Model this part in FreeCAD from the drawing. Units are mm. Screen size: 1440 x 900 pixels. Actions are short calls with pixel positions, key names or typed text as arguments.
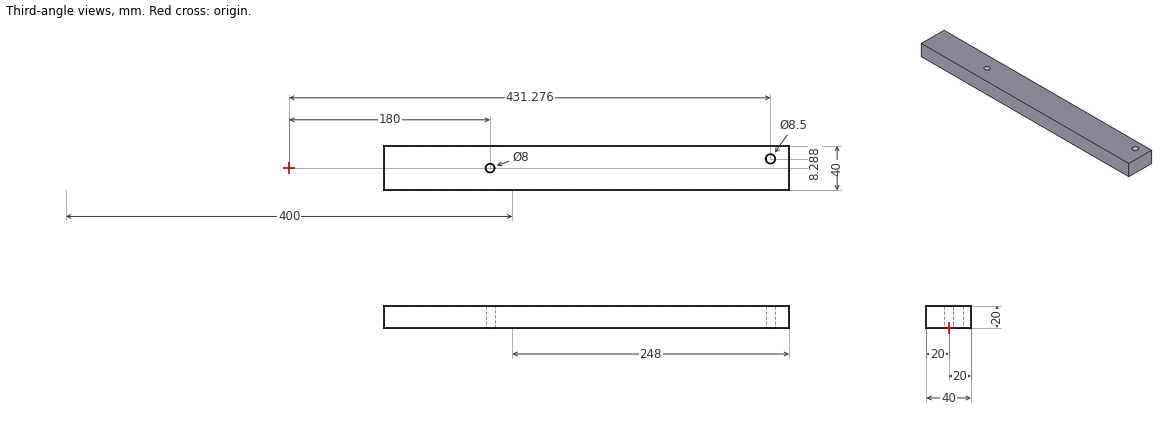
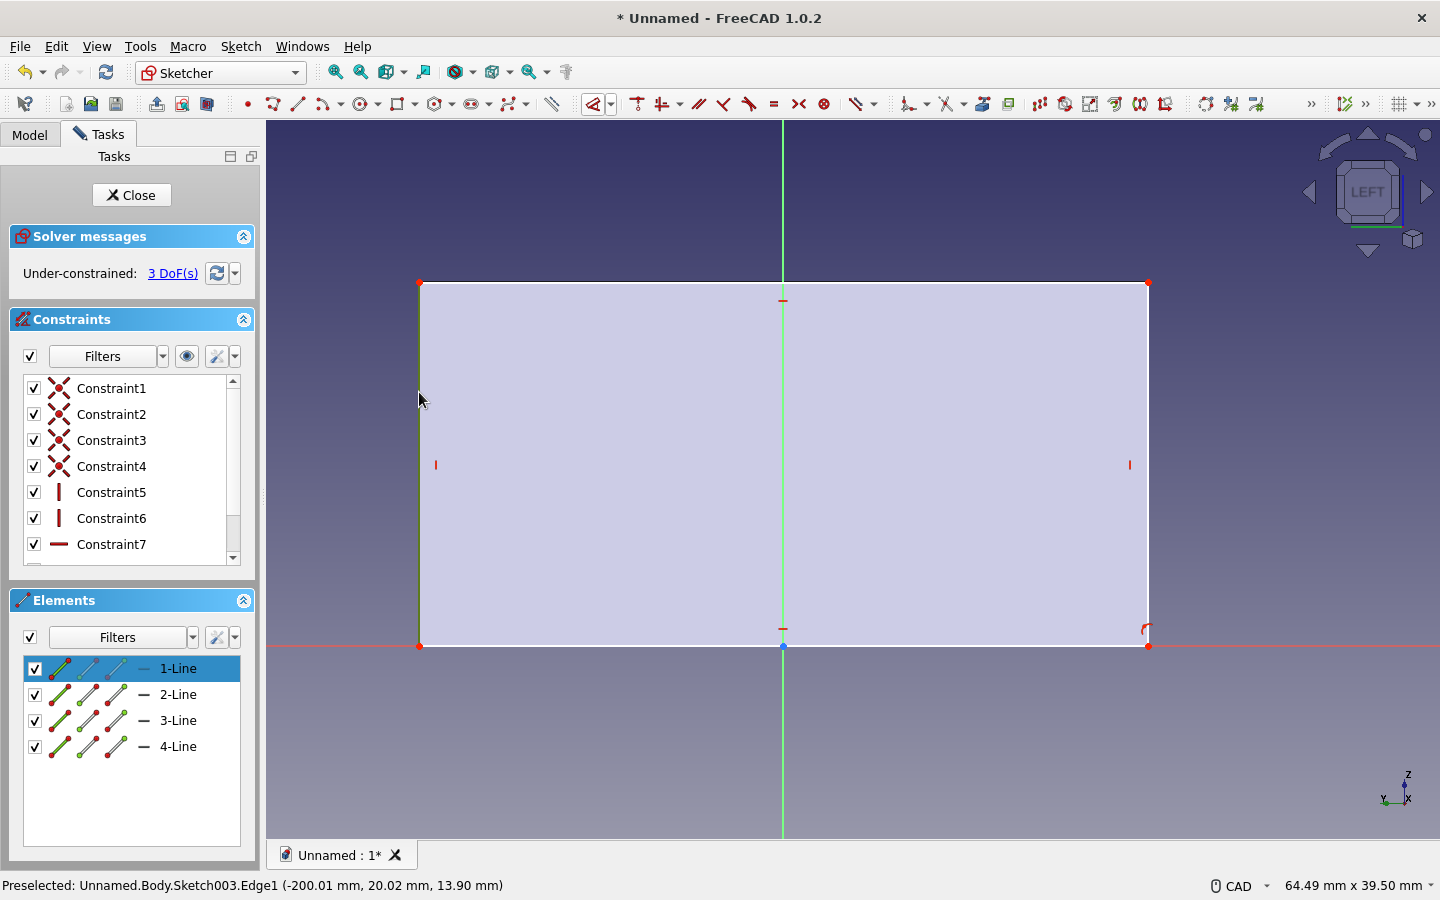
click(610, 104)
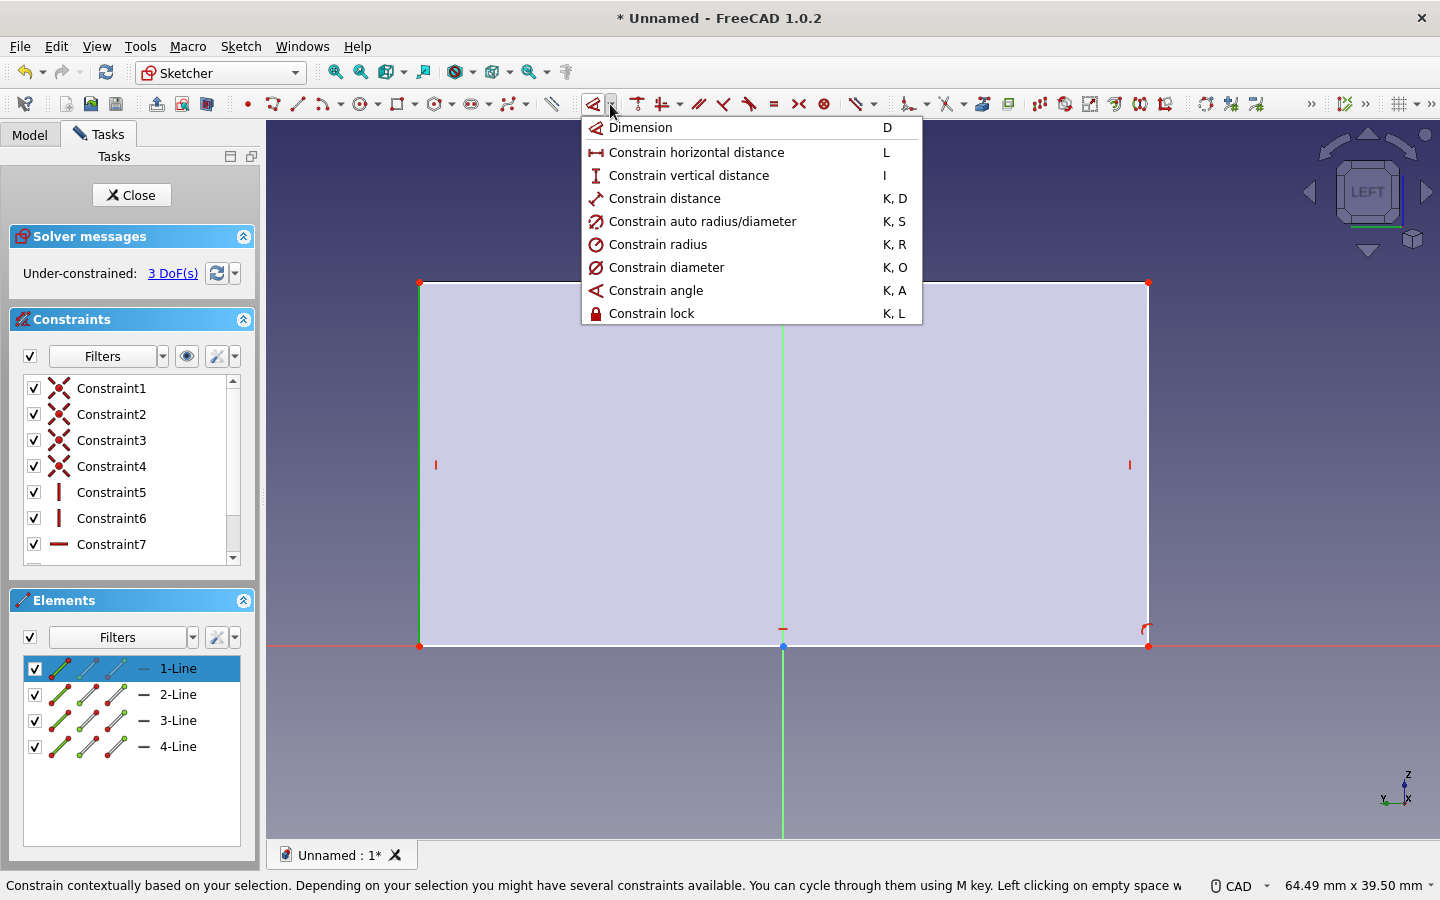
click(752, 176)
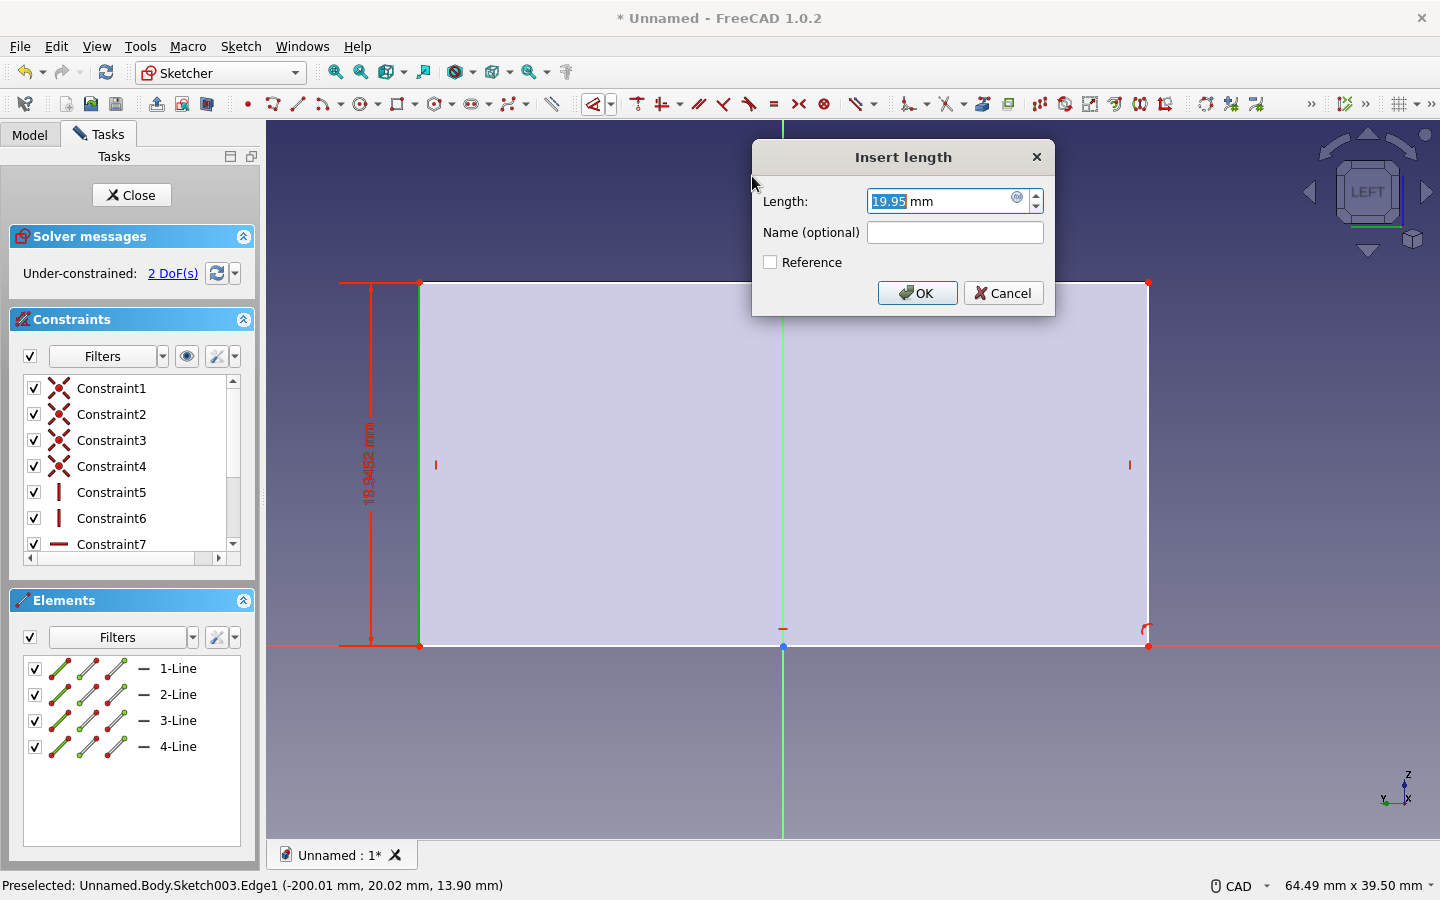
text(20)
key(Return)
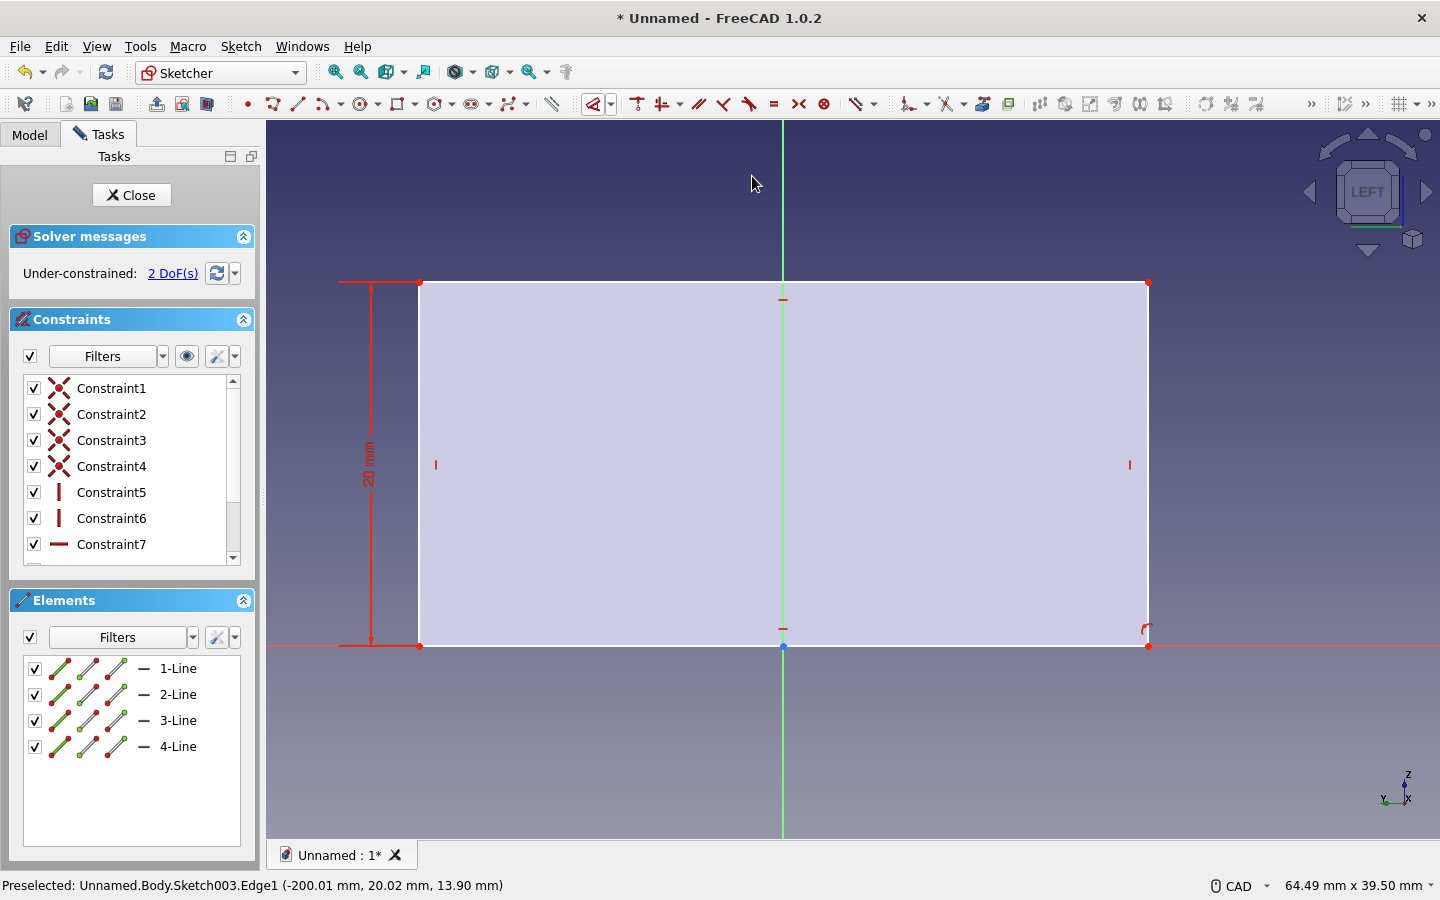
click(638, 646)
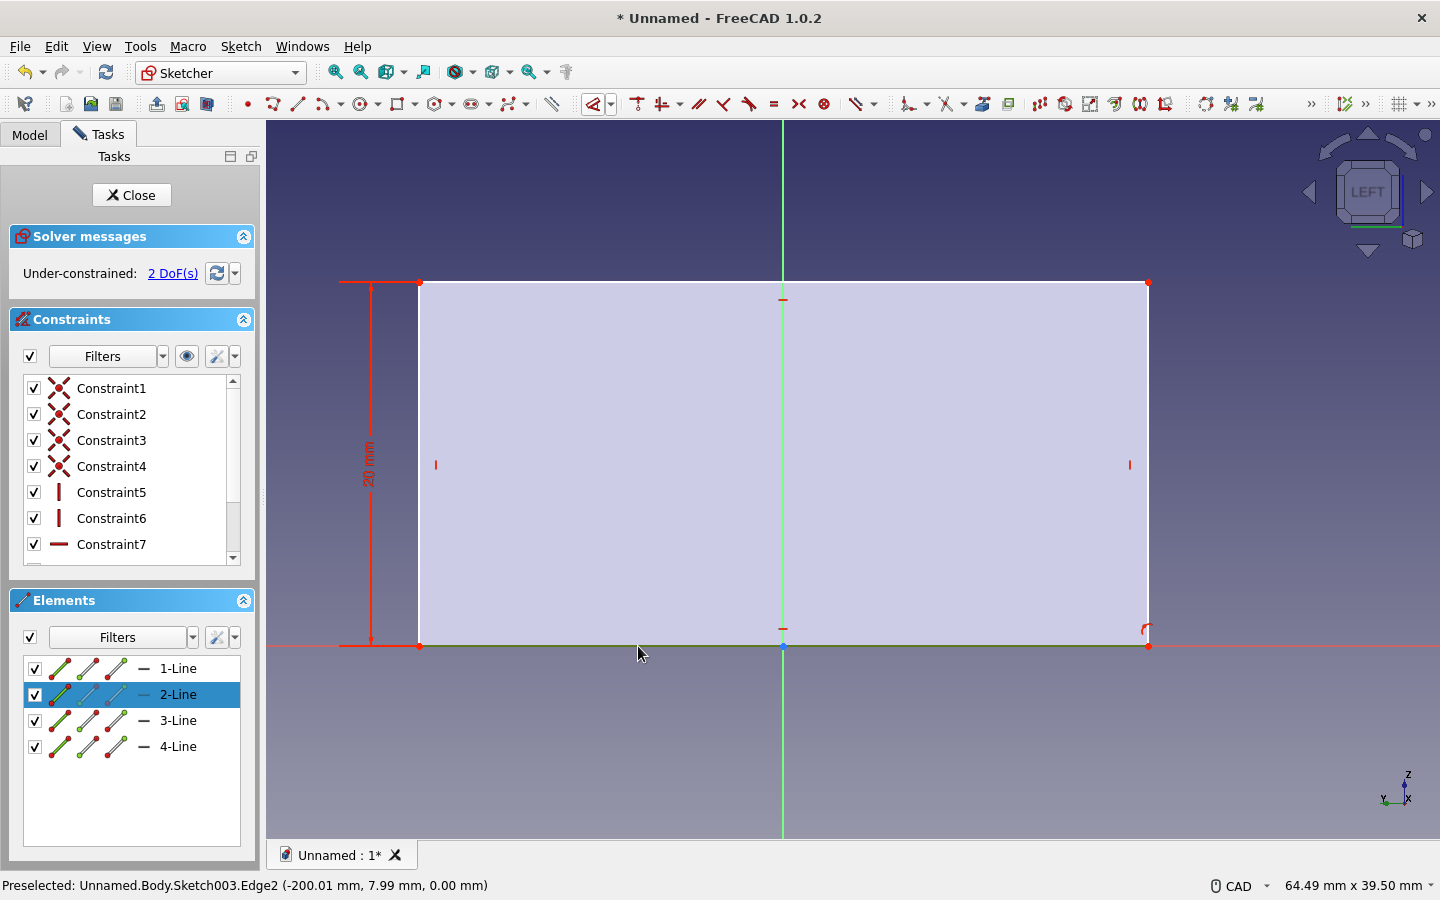
click(610, 104)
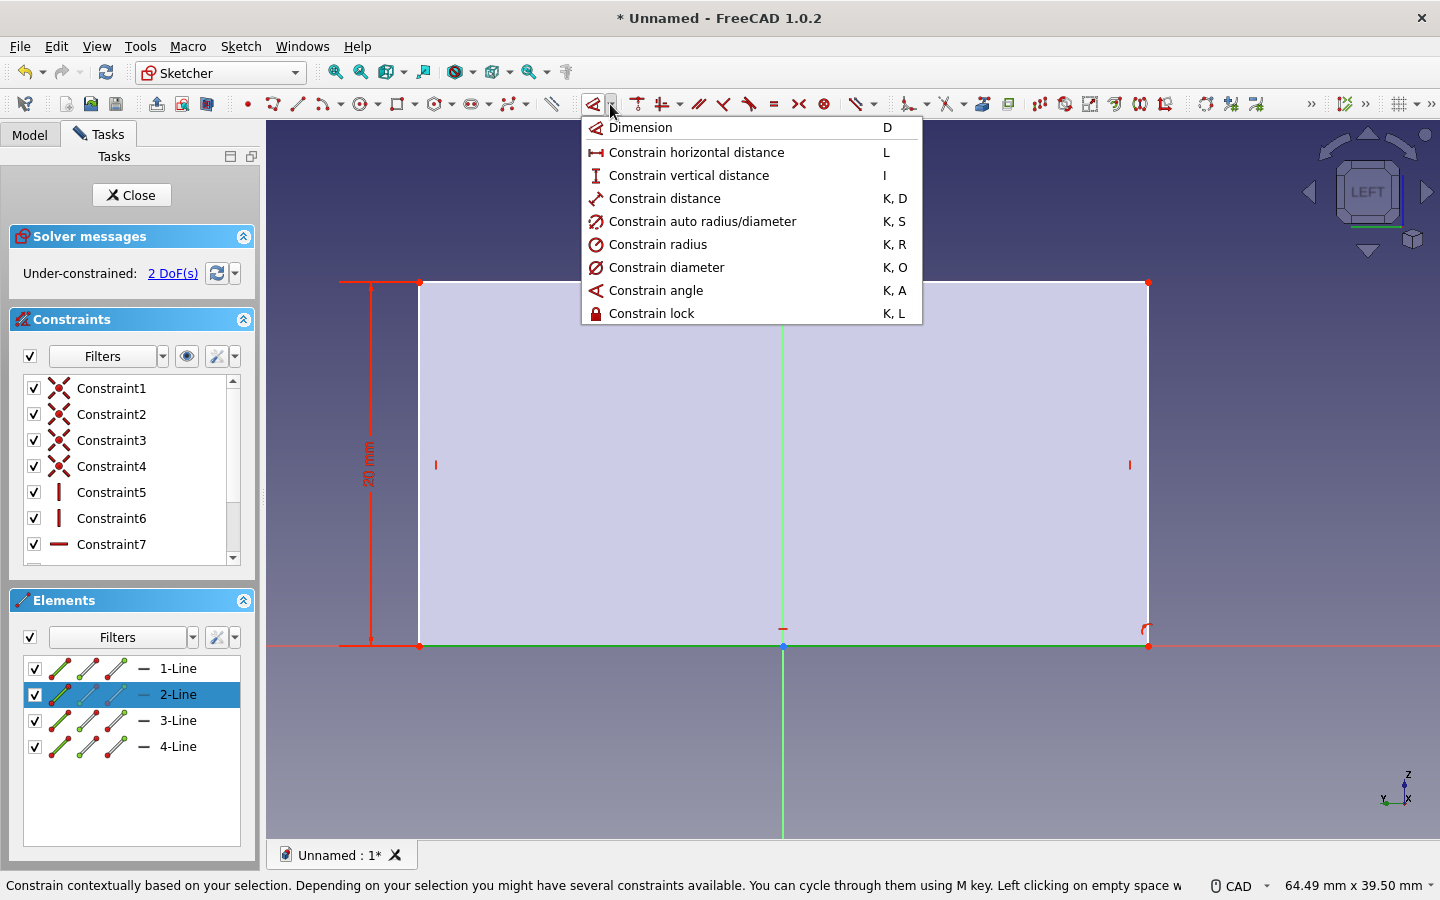
click(752, 152)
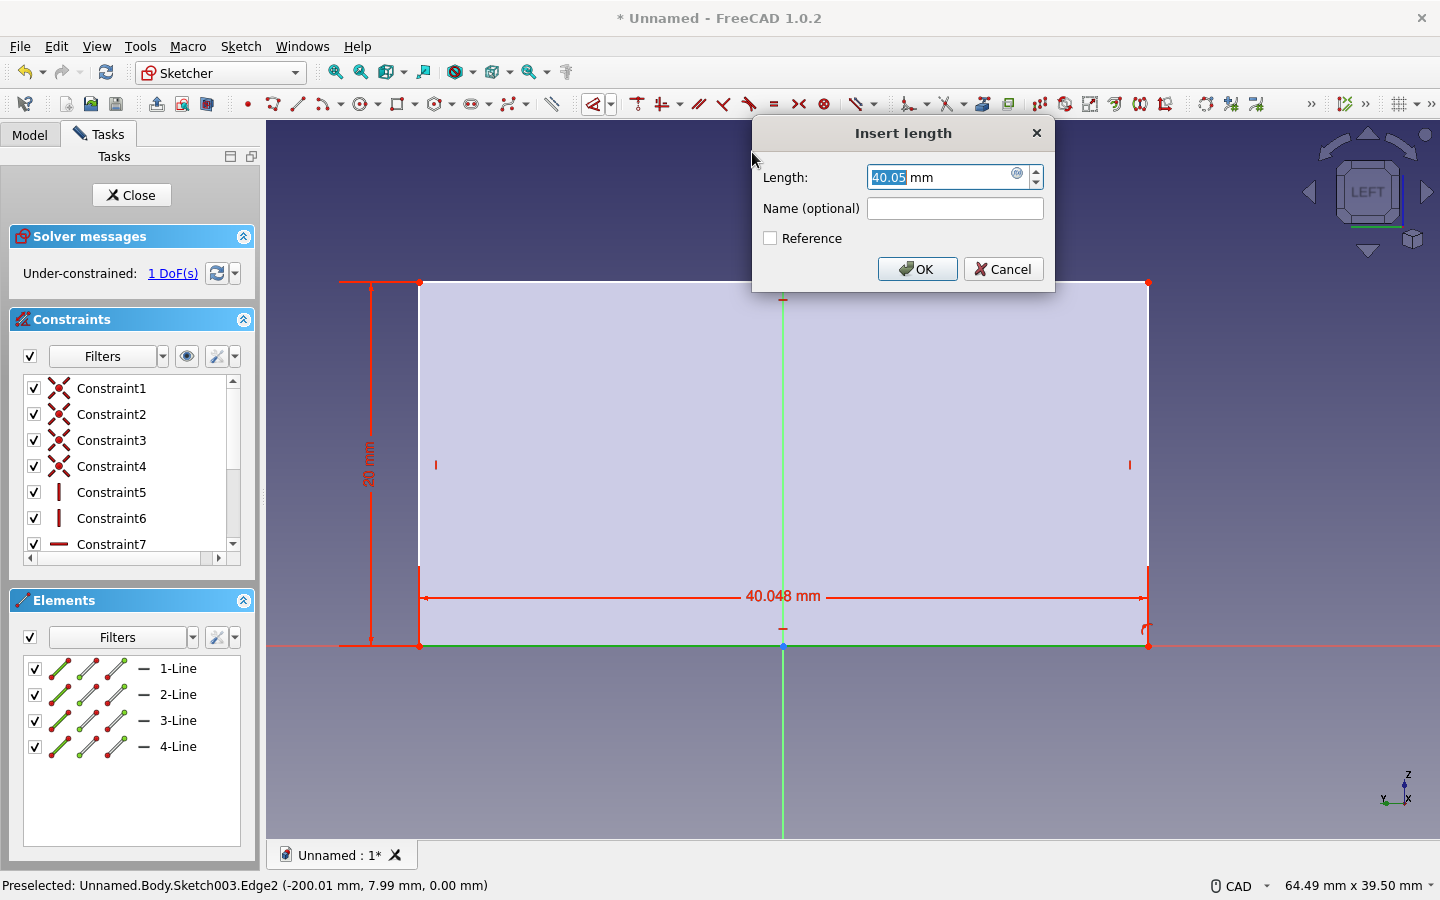
text(40)
key(Return)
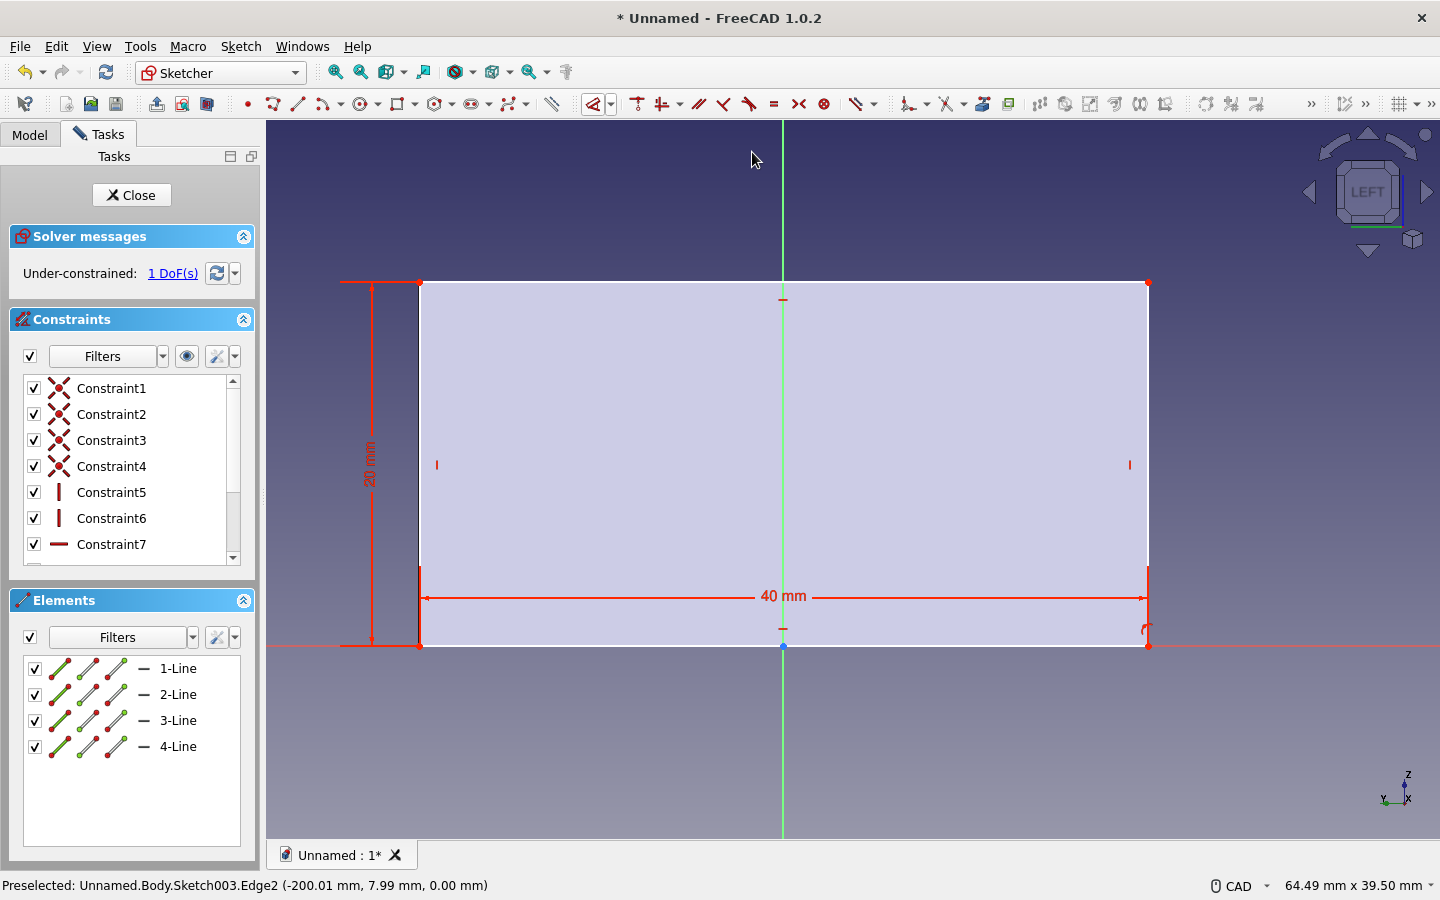
click(420, 282)